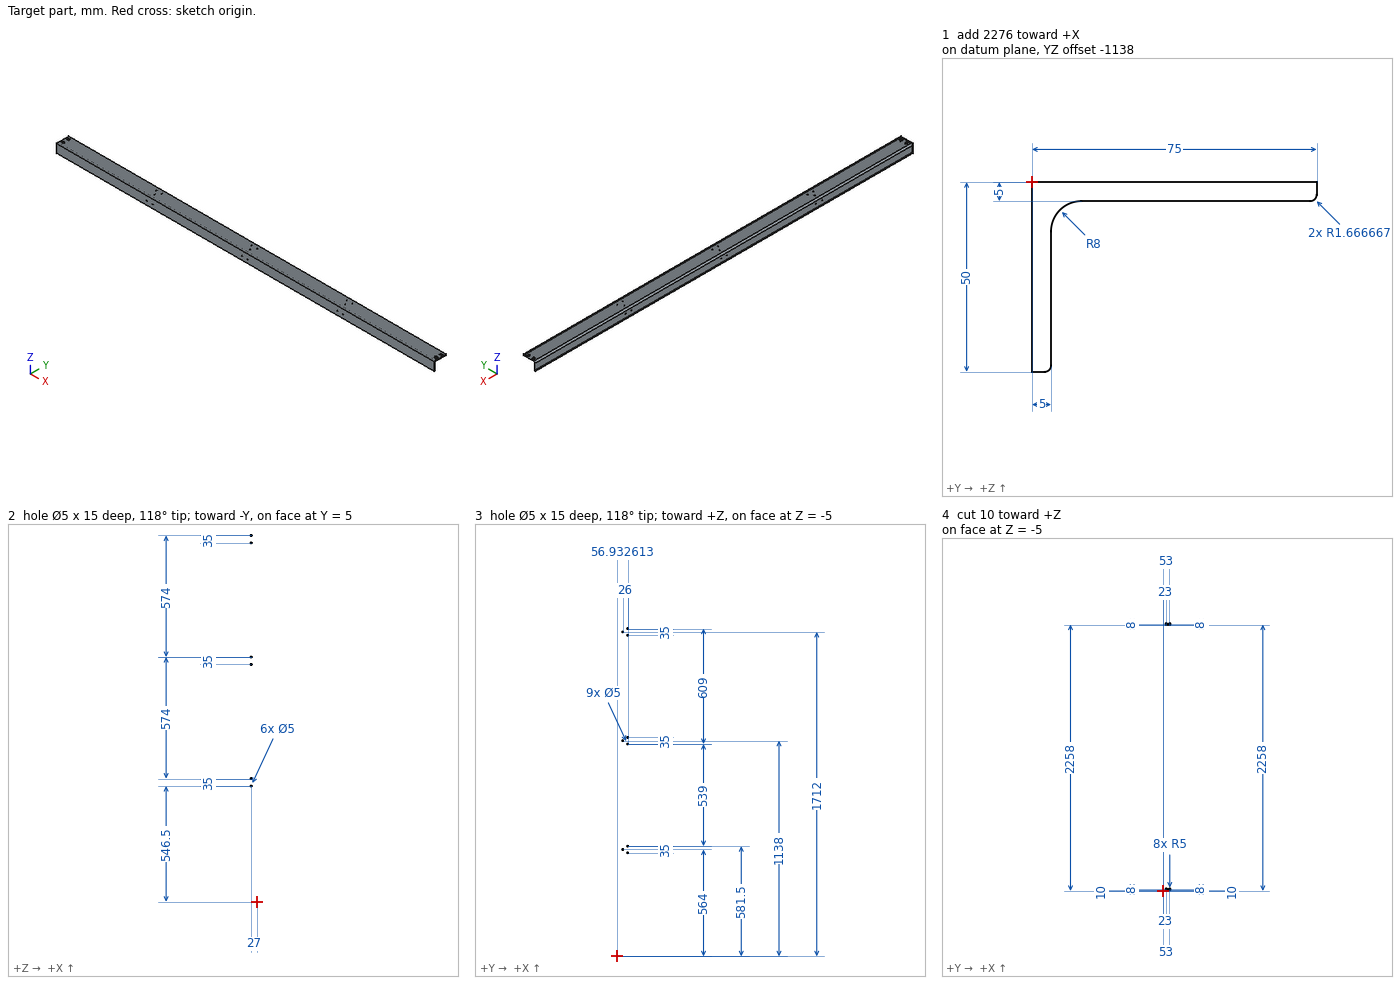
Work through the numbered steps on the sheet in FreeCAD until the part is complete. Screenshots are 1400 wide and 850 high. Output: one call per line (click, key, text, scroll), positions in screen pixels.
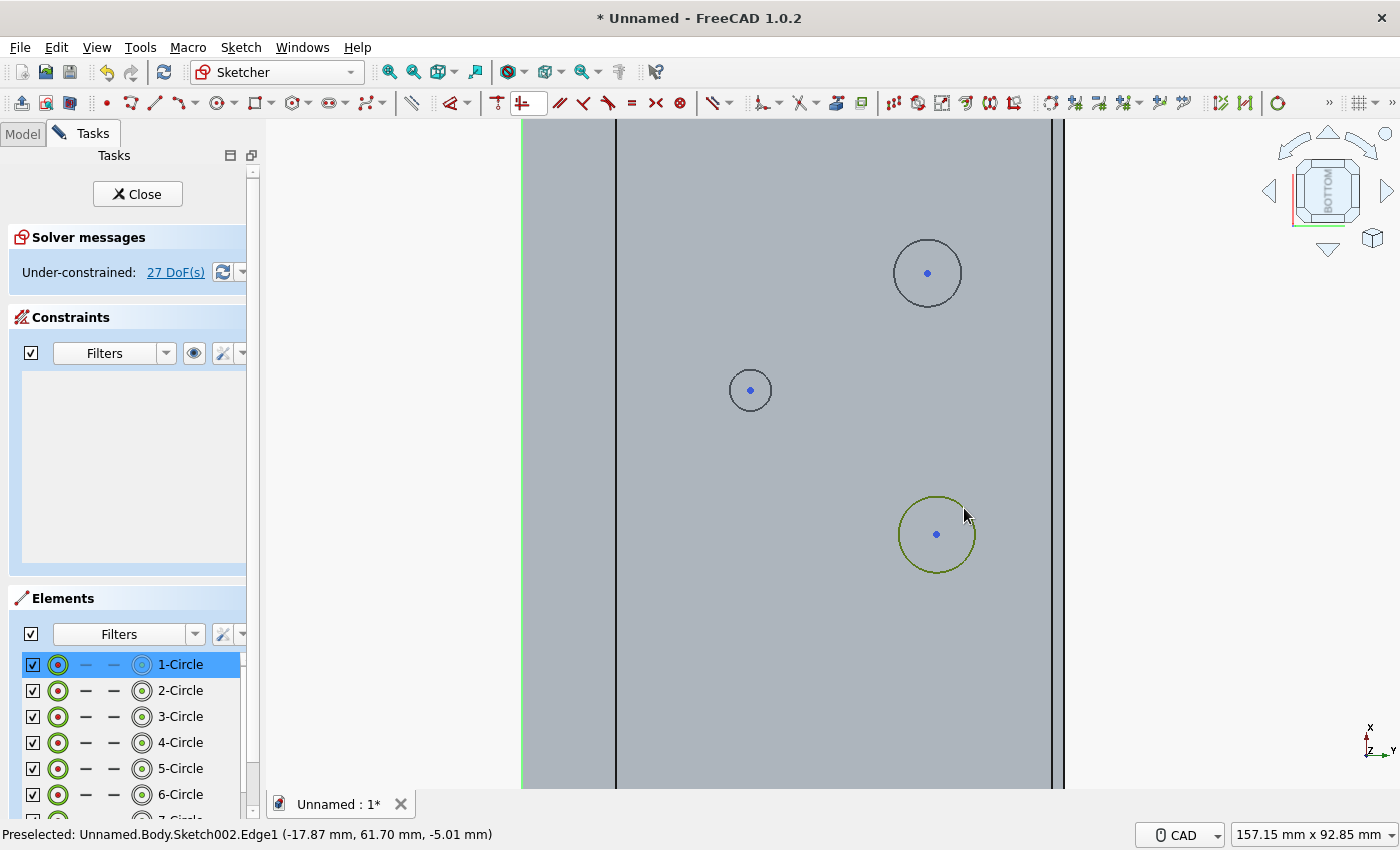
scroll(766, 374, down, 16)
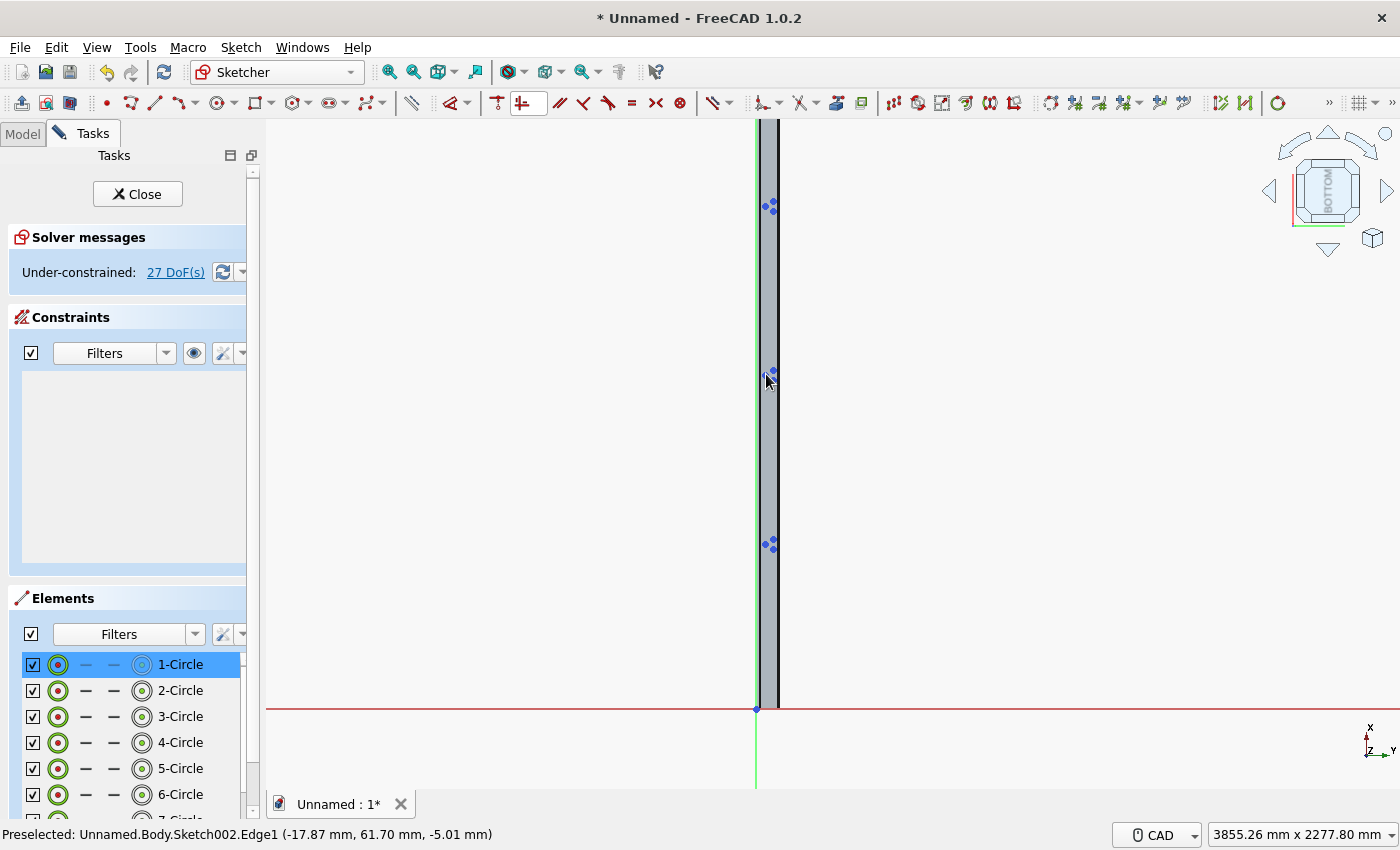
scroll(775, 201, up, 11)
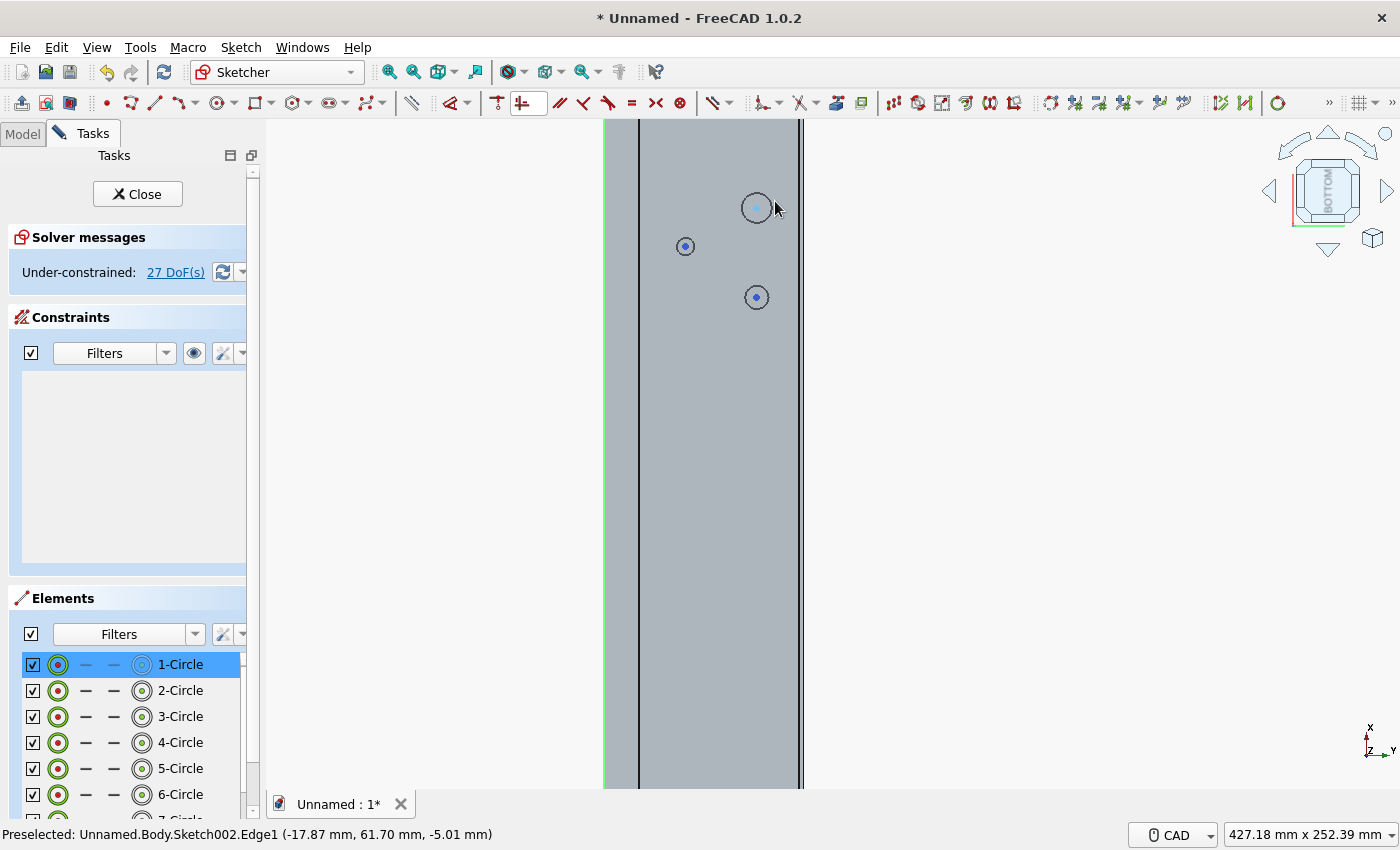
click(767, 197)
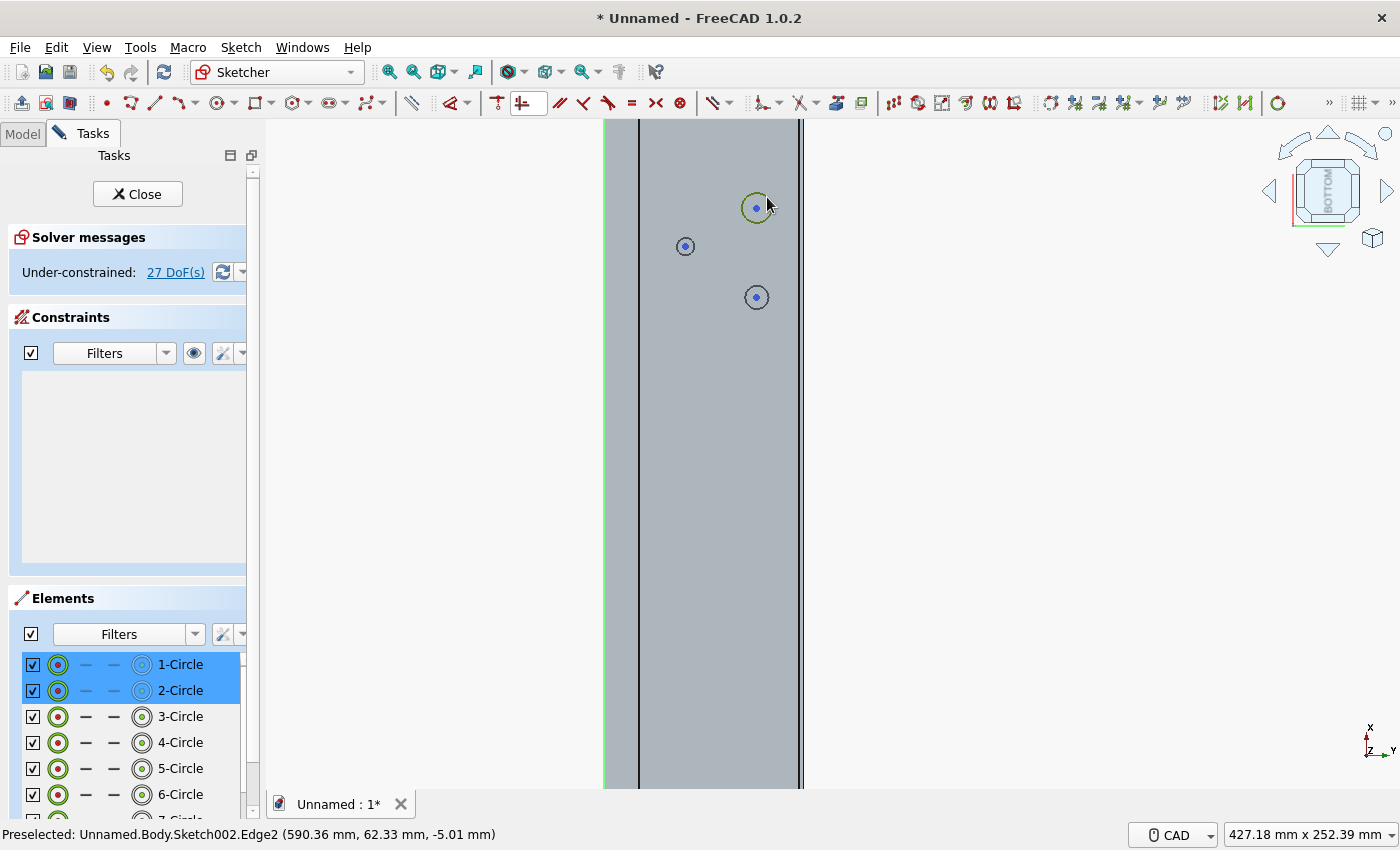
click(765, 289)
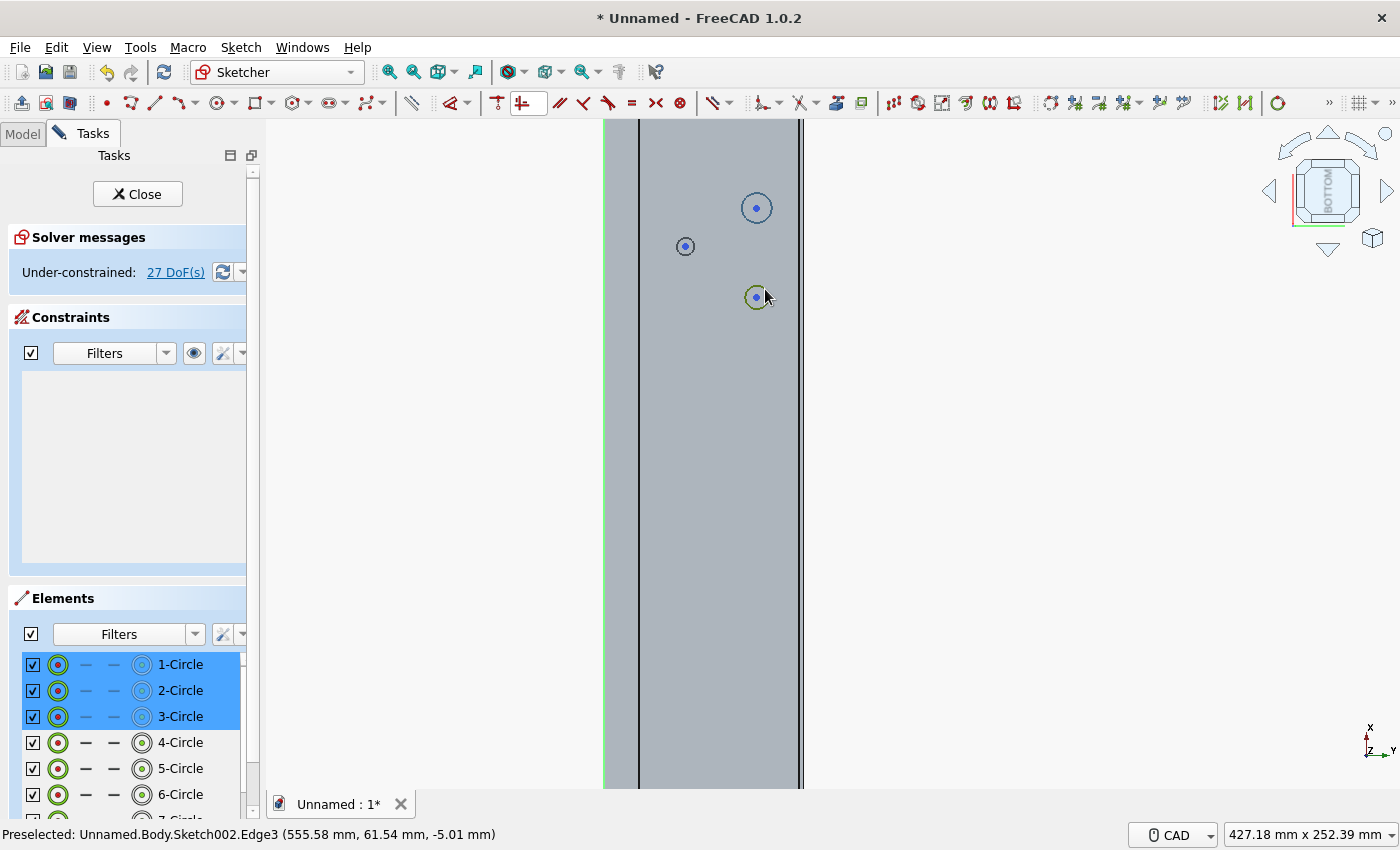
scroll(692, 240, up, 2)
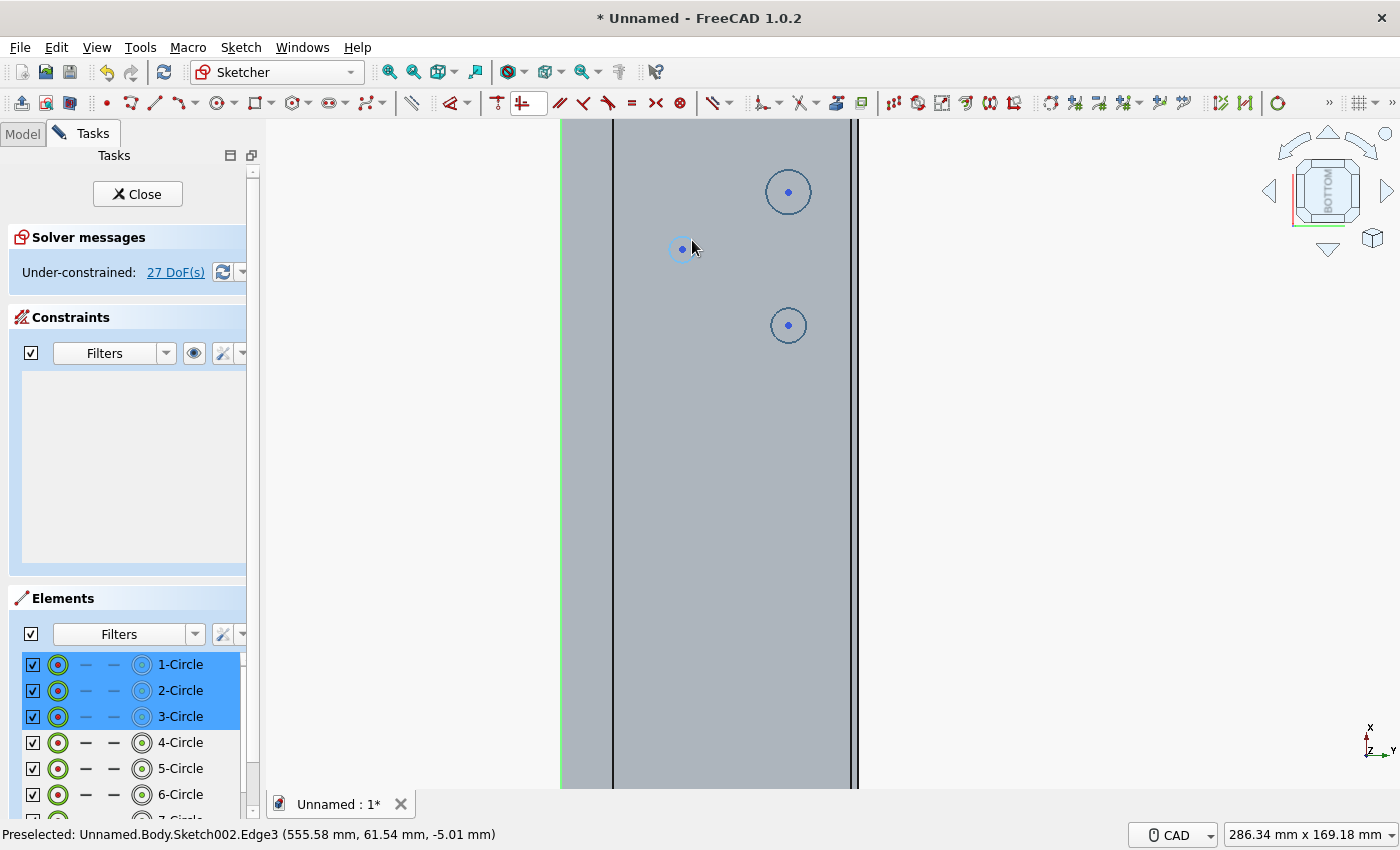
click(691, 241)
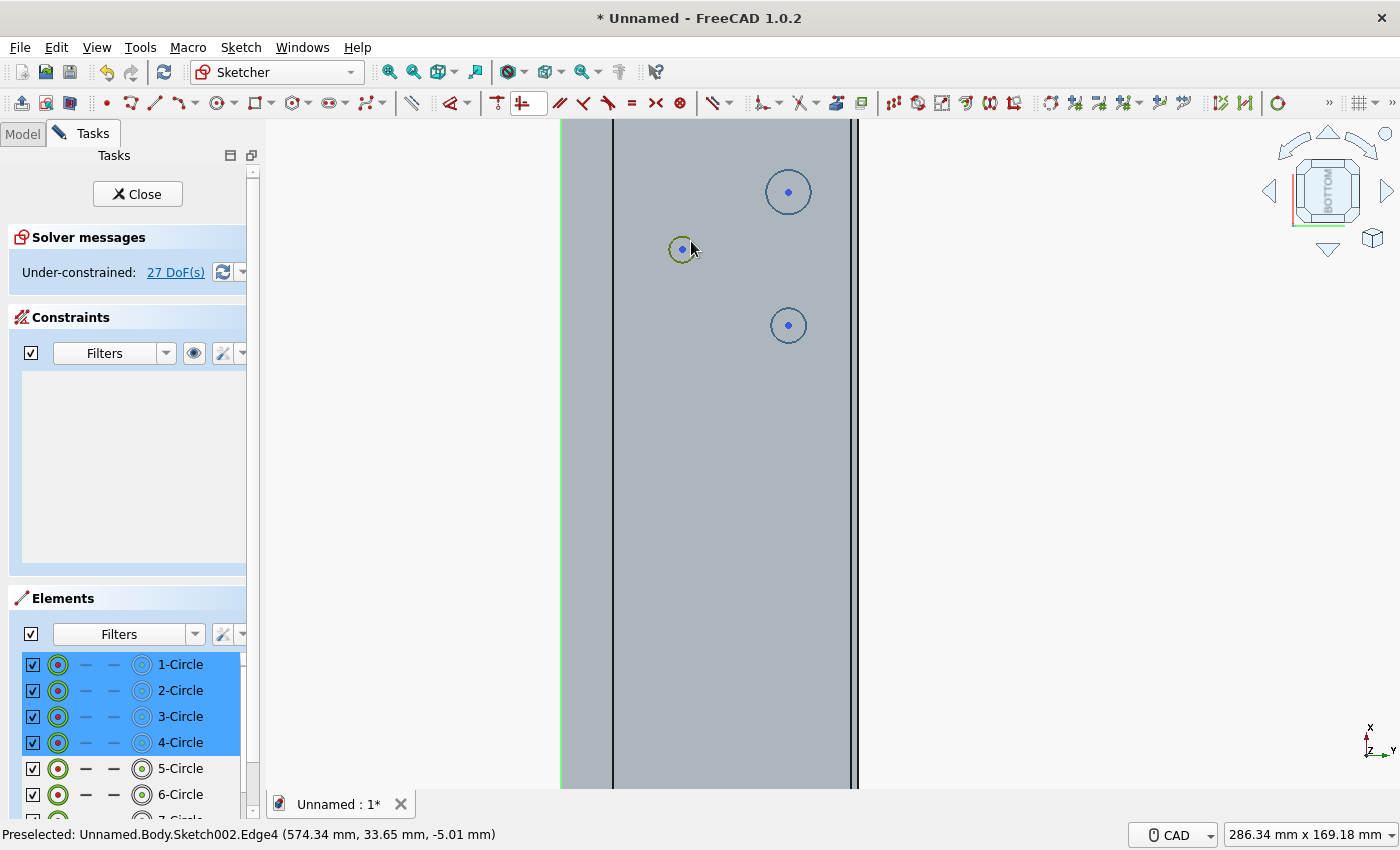
scroll(770, 251, down, 14)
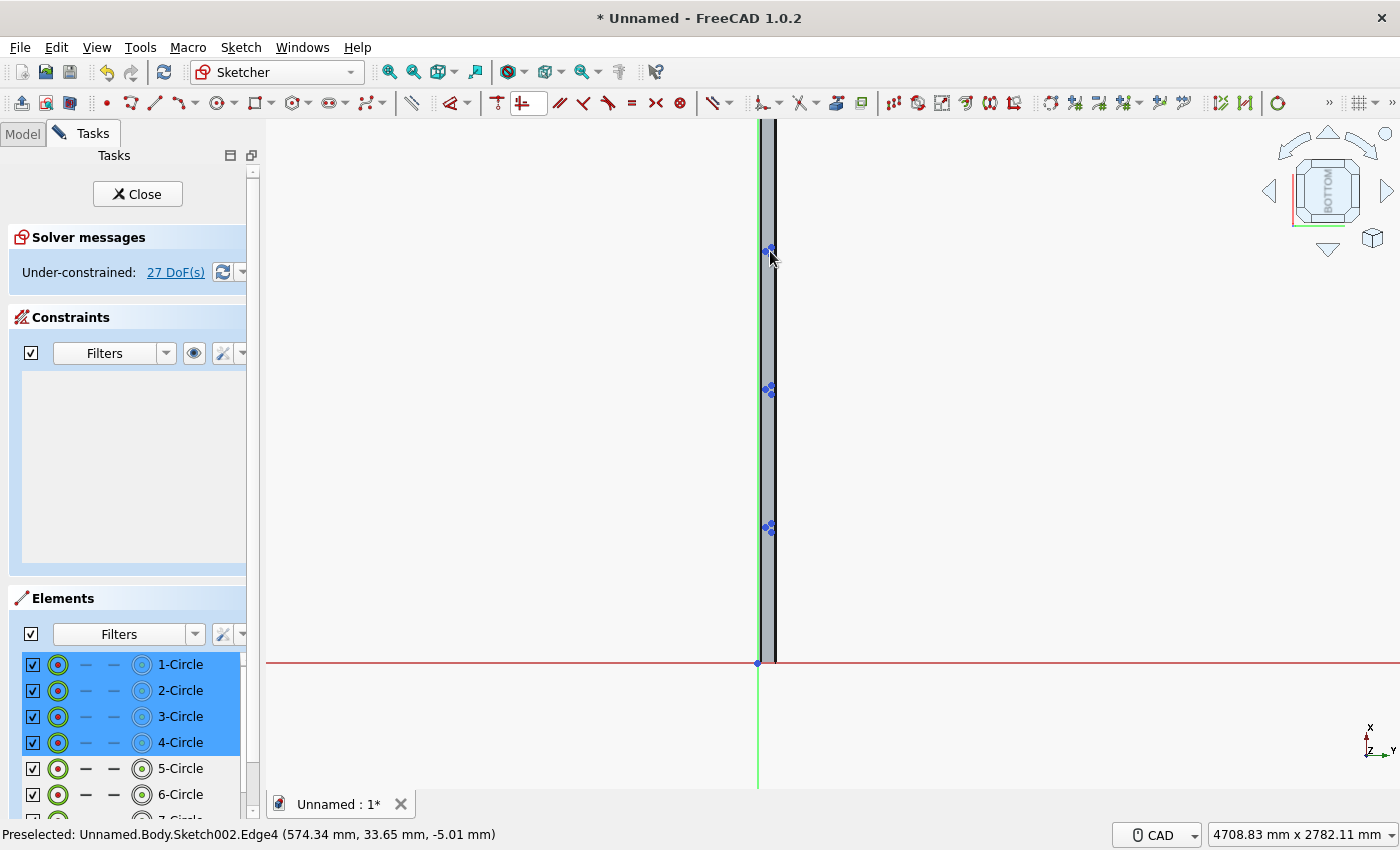
scroll(773, 523, up, 13)